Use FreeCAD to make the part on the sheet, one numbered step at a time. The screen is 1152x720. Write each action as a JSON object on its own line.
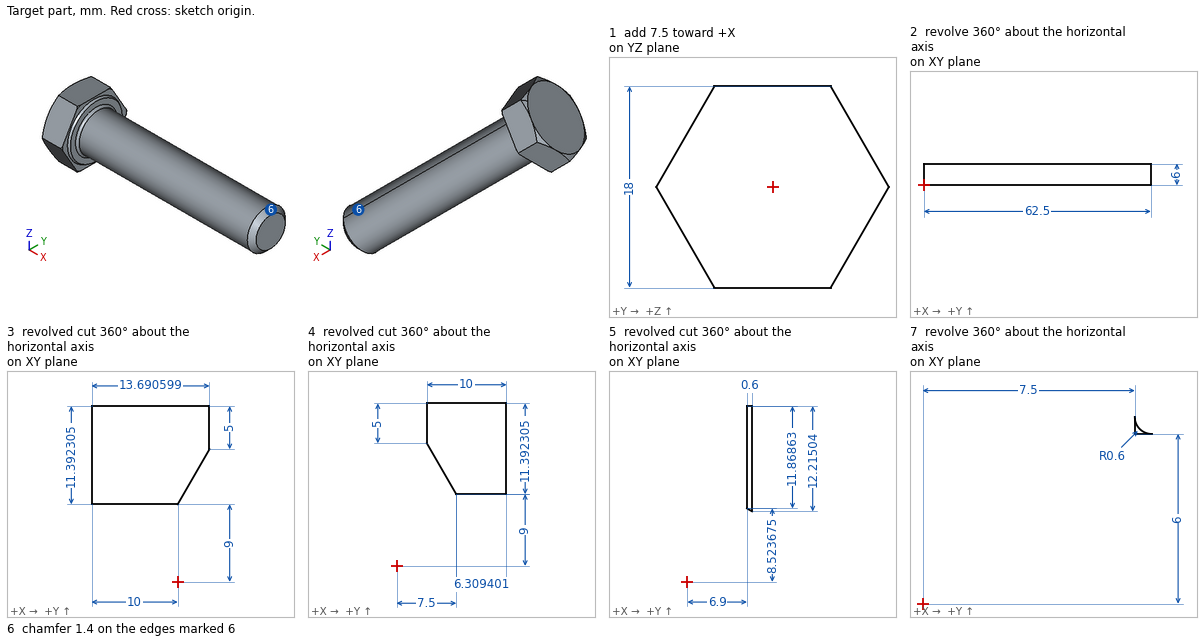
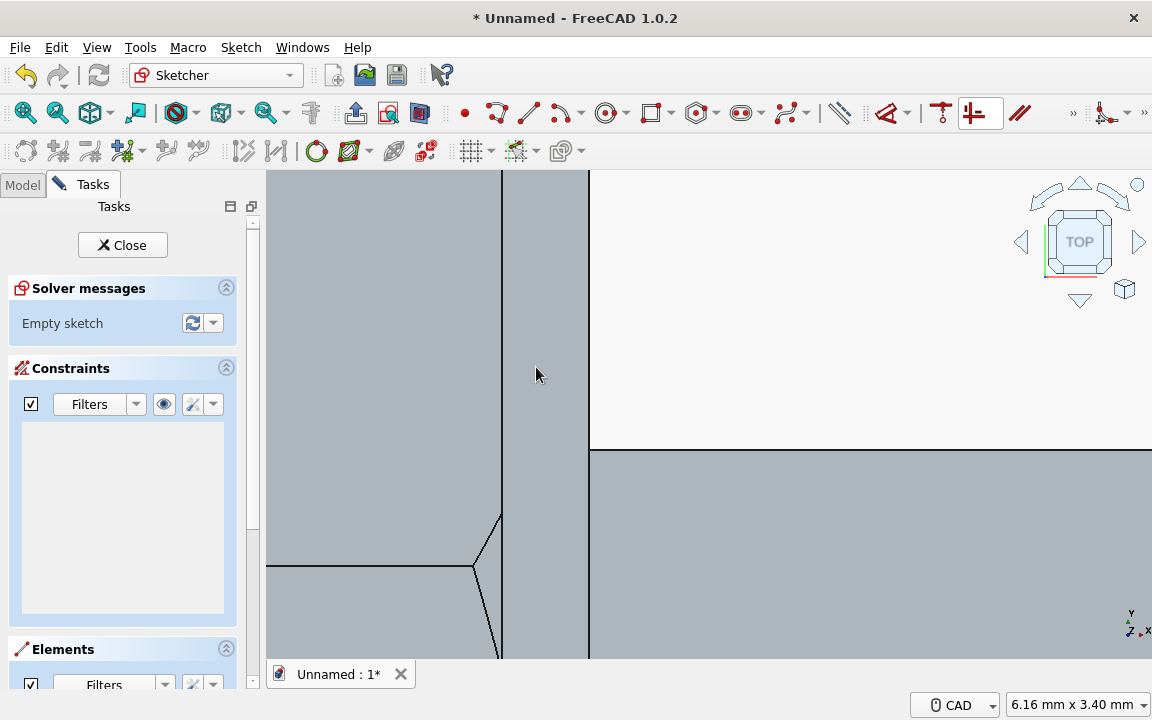
{"action": "scroll", "coordinate": [628, 404], "scroll_direction": "up", "scroll_amount": 6}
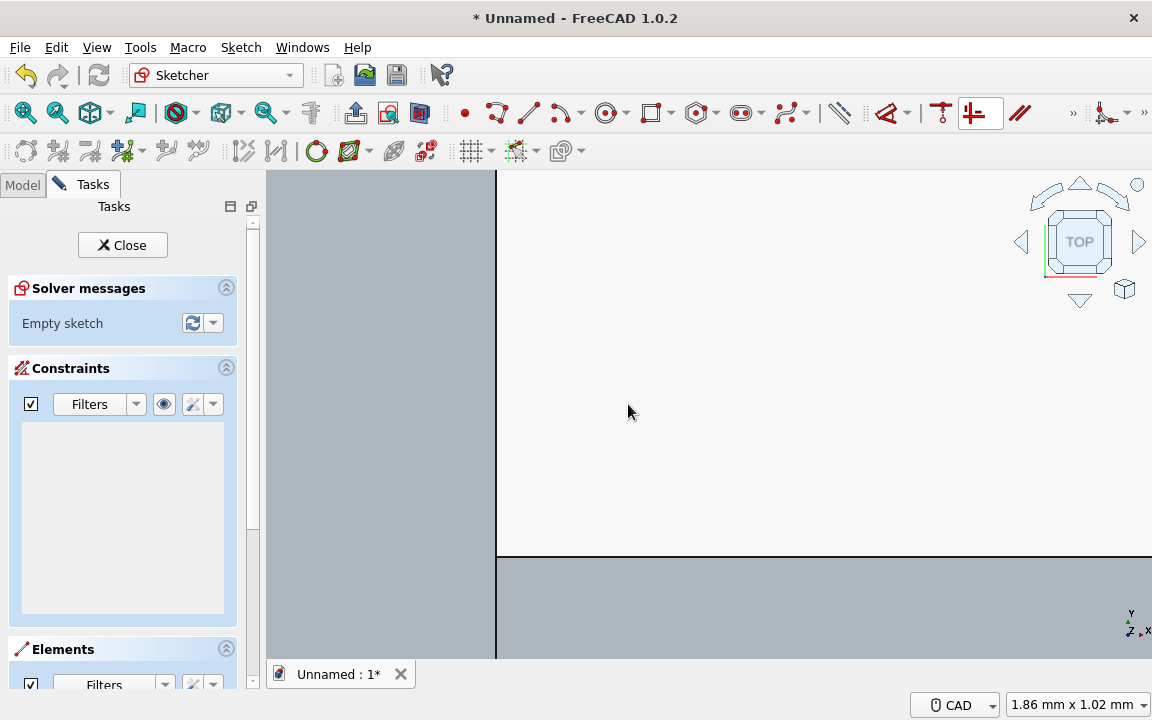
{"action": "left_click", "coordinate": [498, 114]}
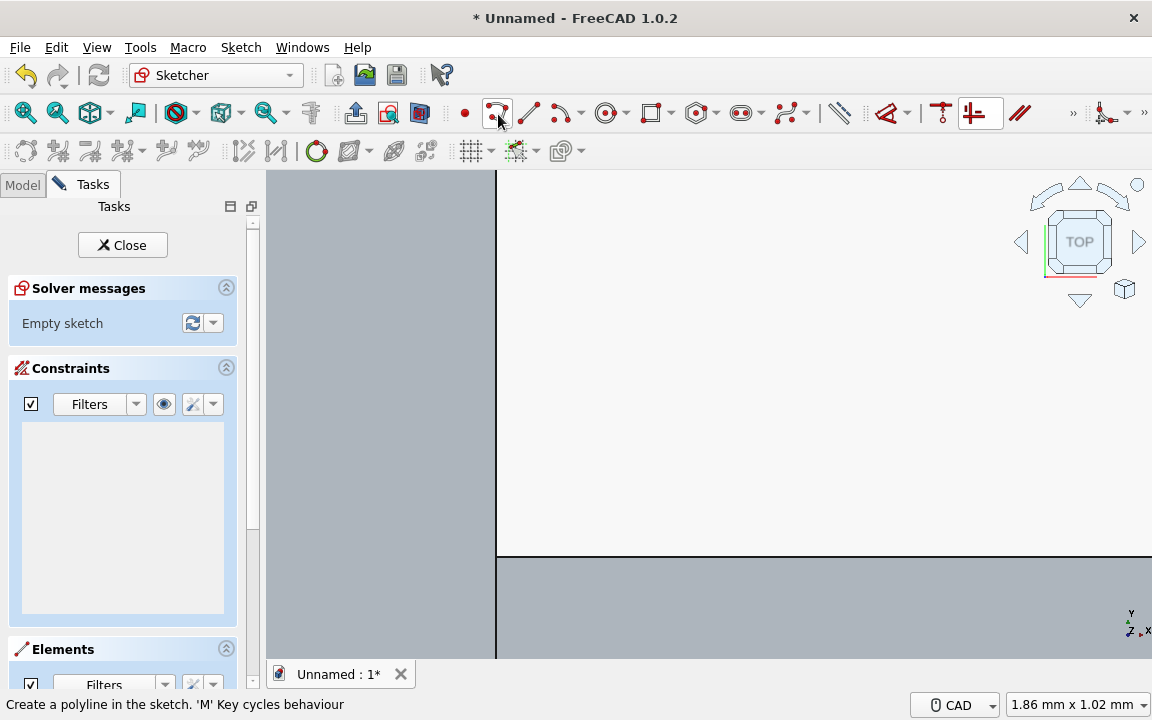
{"action": "left_click", "coordinate": [496, 270]}
{"action": "left_click", "coordinate": [496, 557]}
{"action": "left_click", "coordinate": [783, 557]}
{"action": "right_click", "coordinate": [783, 557]}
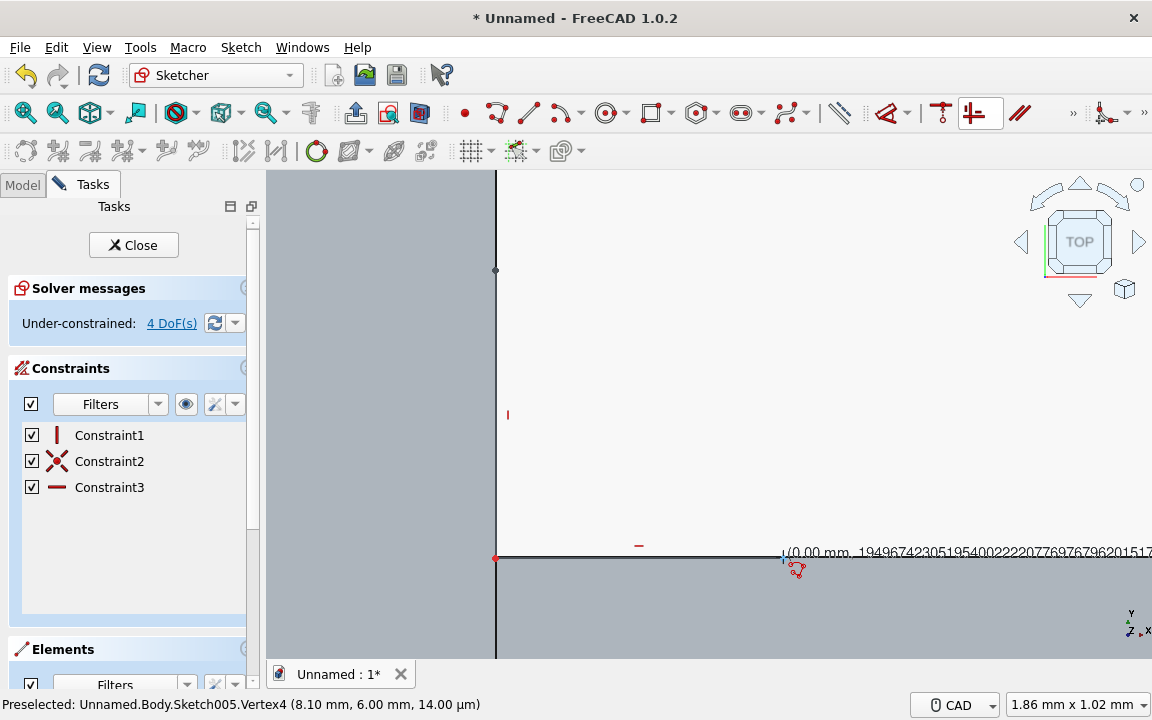
{"action": "left_click", "coordinate": [584, 114]}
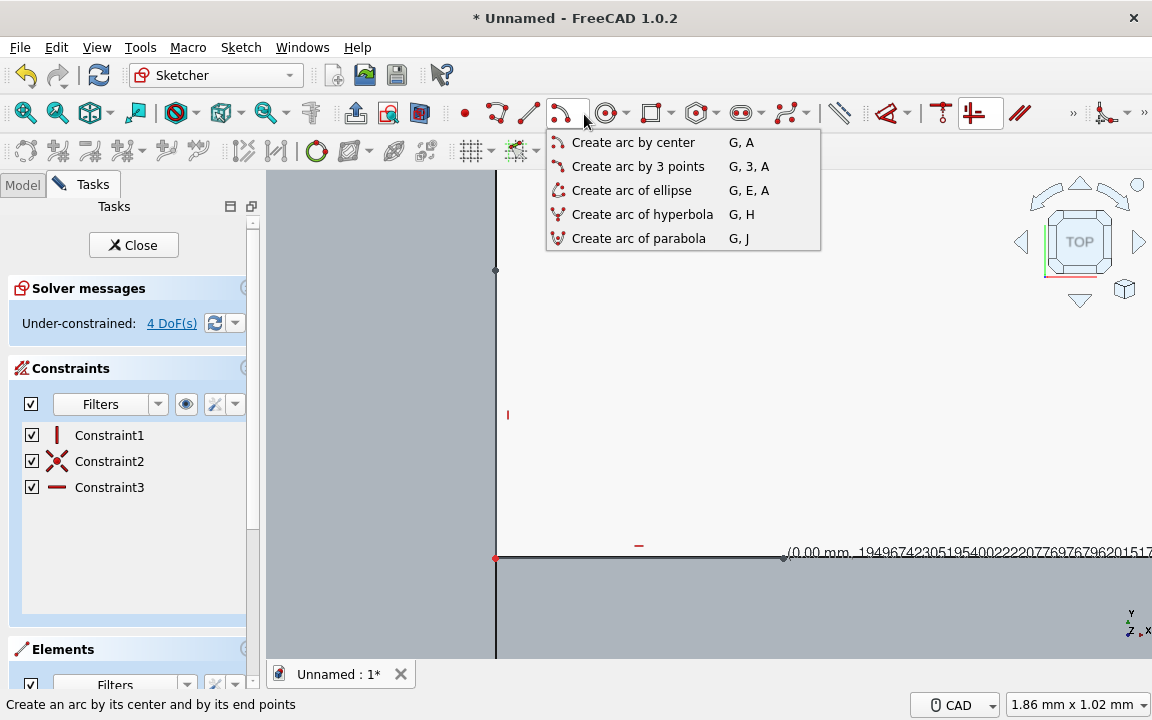
{"action": "left_click", "coordinate": [684, 166]}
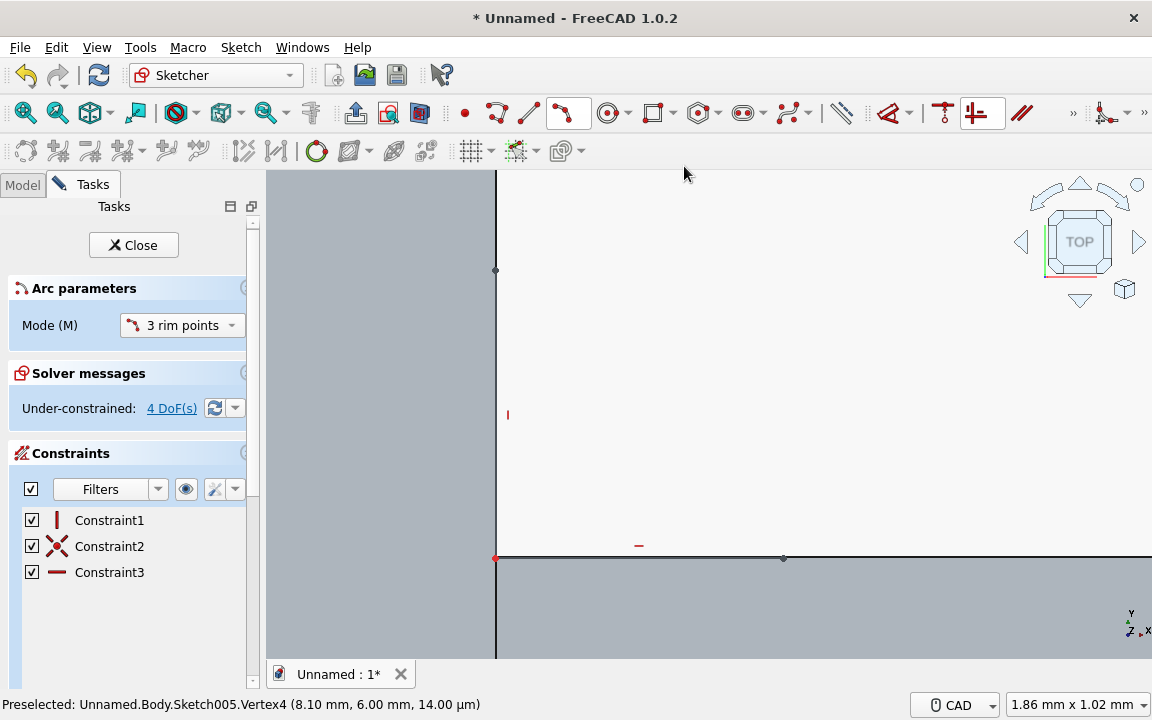
{"action": "left_click", "coordinate": [783, 558]}
{"action": "left_click", "coordinate": [496, 271]}
{"action": "left_click", "coordinate": [580, 473]}
{"action": "key", "text": "Escape"}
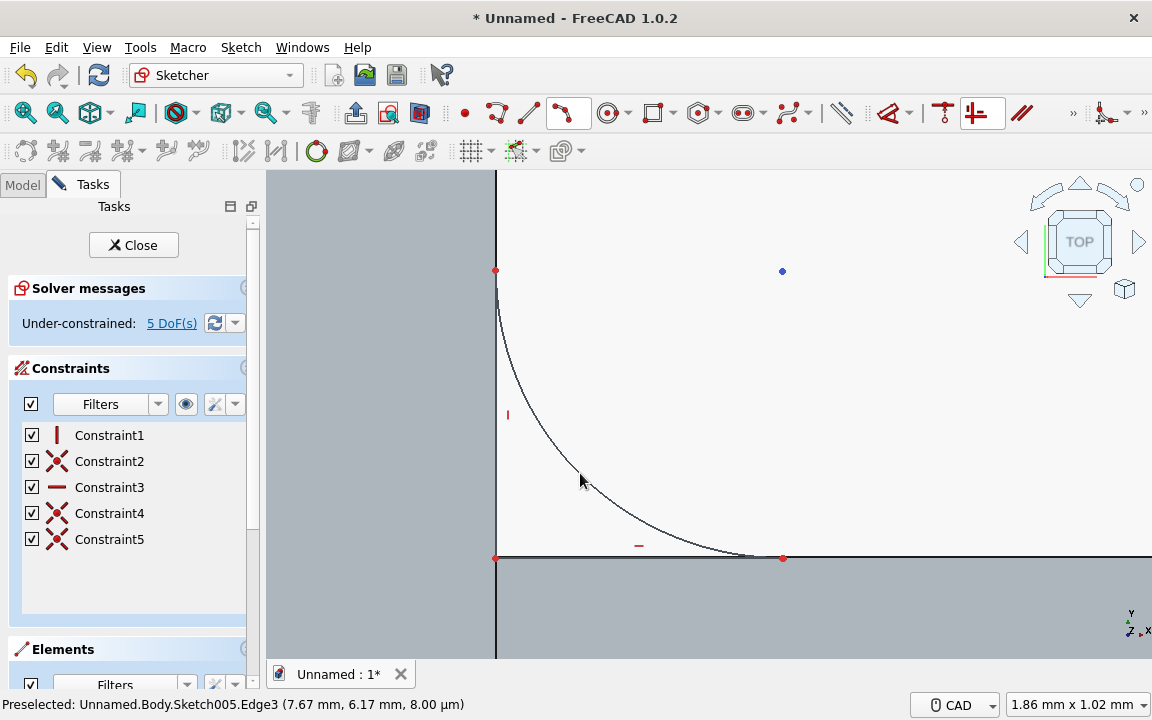
{"action": "left_click", "coordinate": [496, 357]}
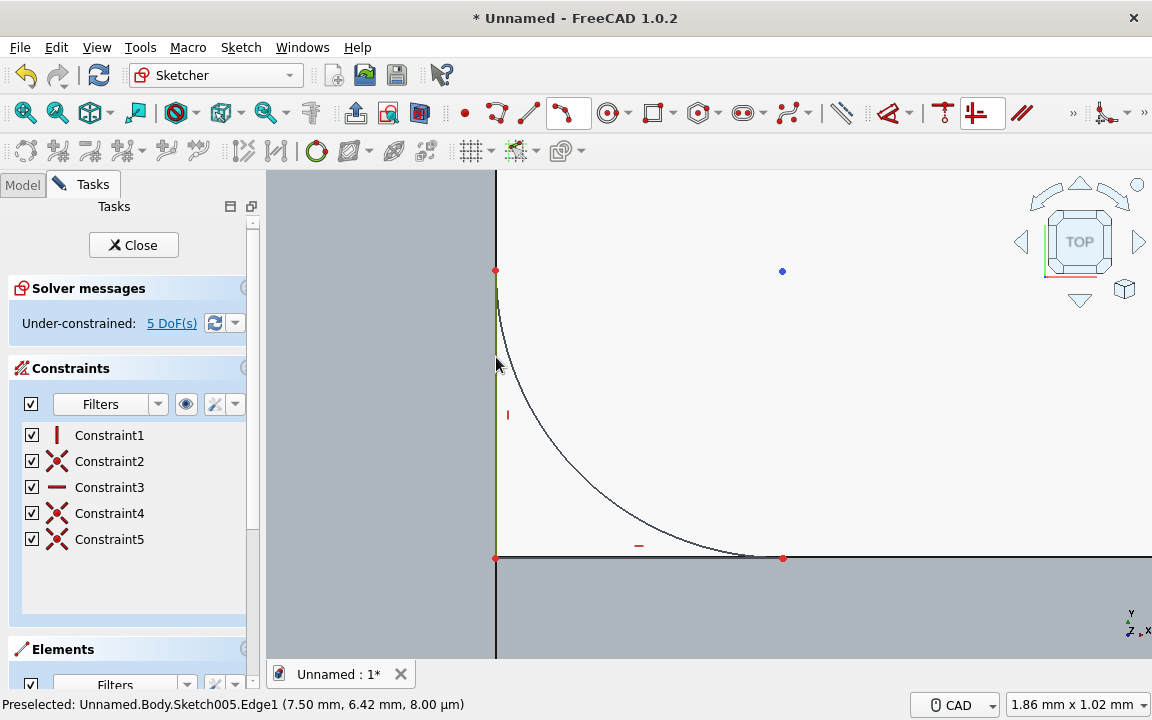
{"action": "left_click", "coordinate": [527, 401]}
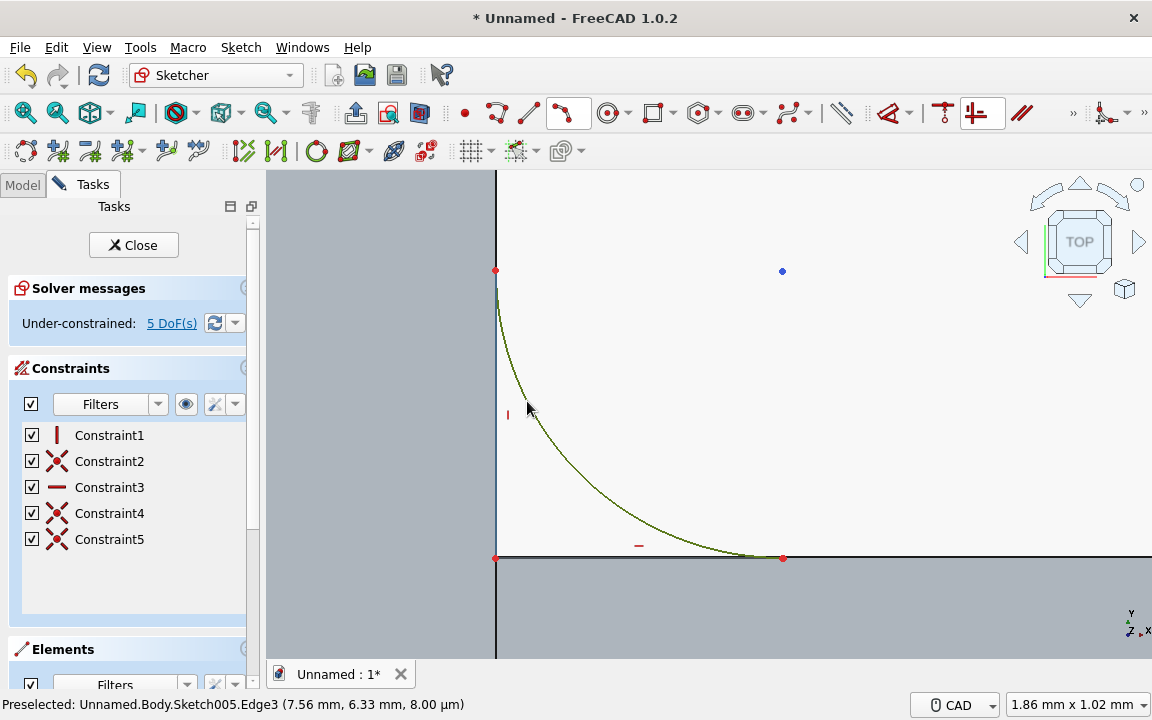
{"action": "key", "text": "t"}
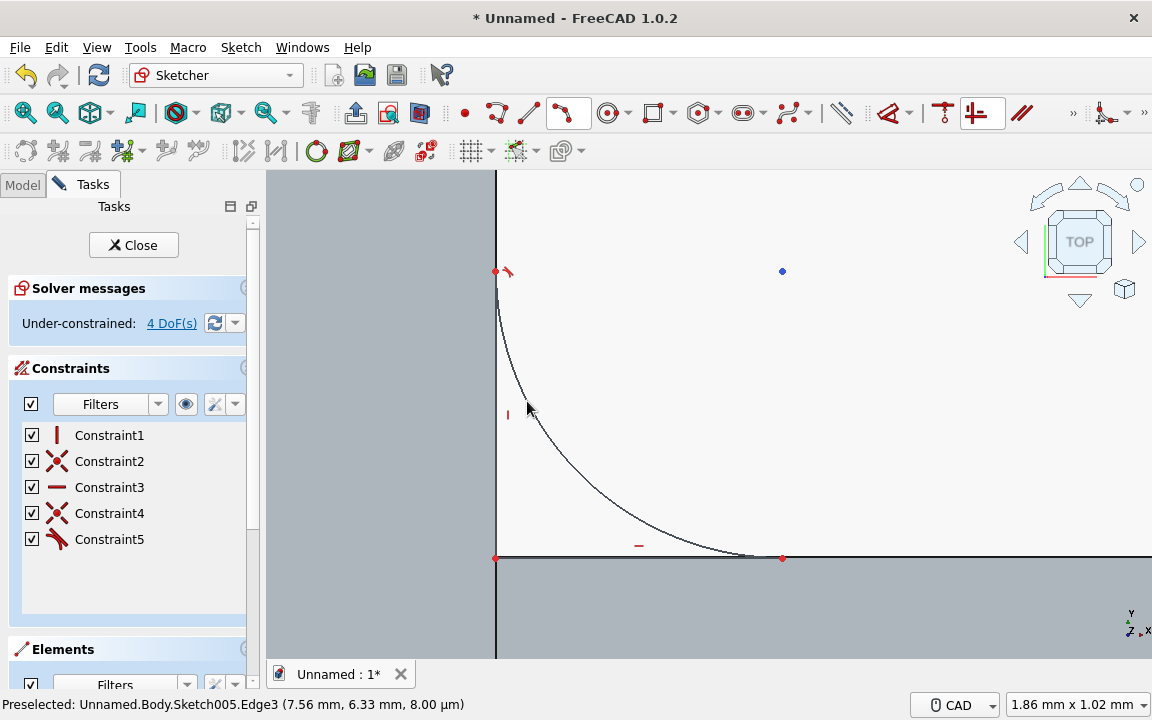
{"action": "left_click", "coordinate": [582, 558]}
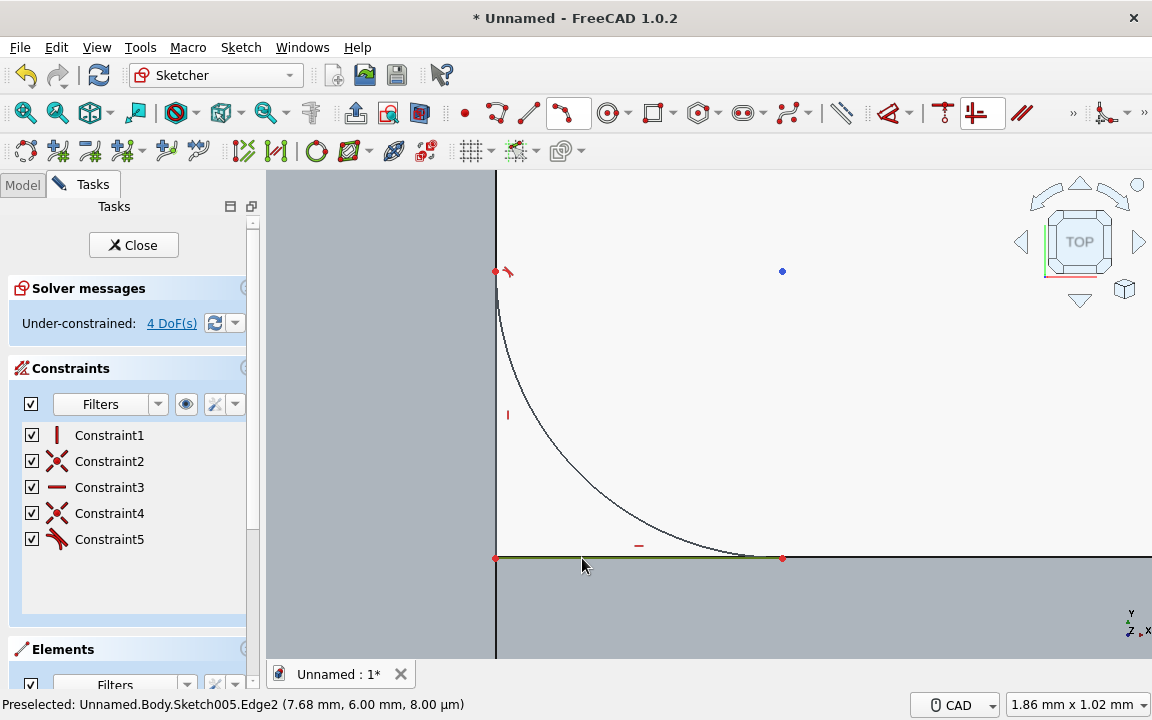
{"action": "left_click", "coordinate": [527, 401]}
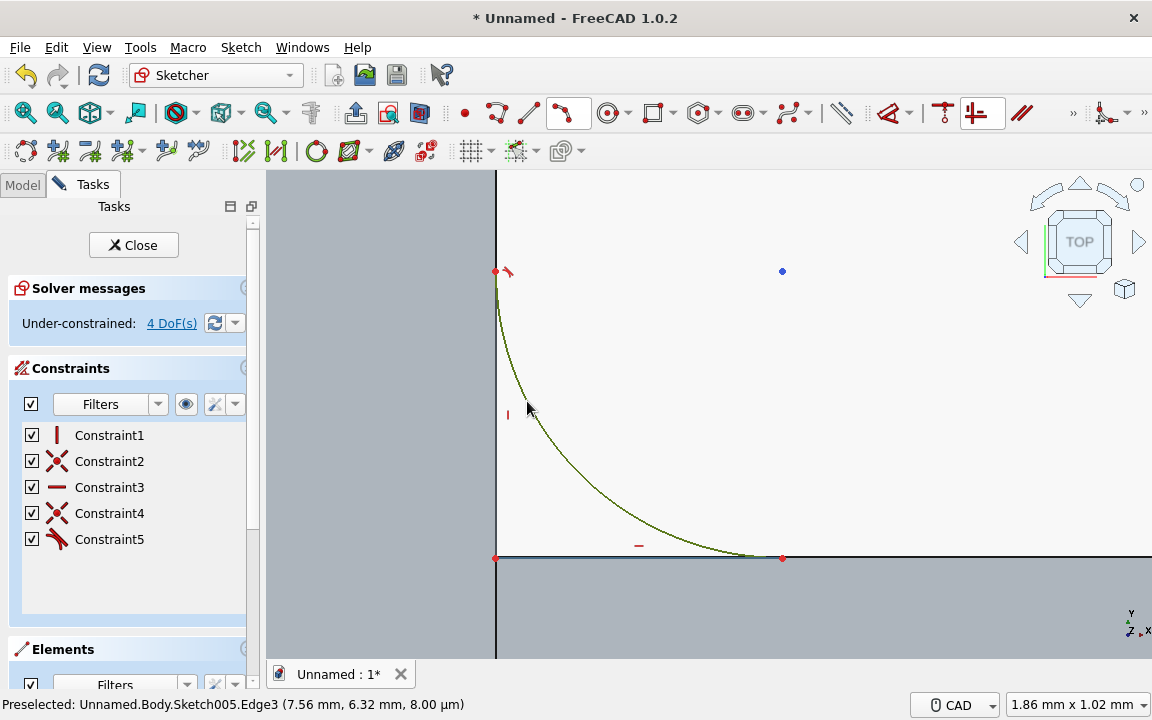
{"action": "key", "text": "t"}